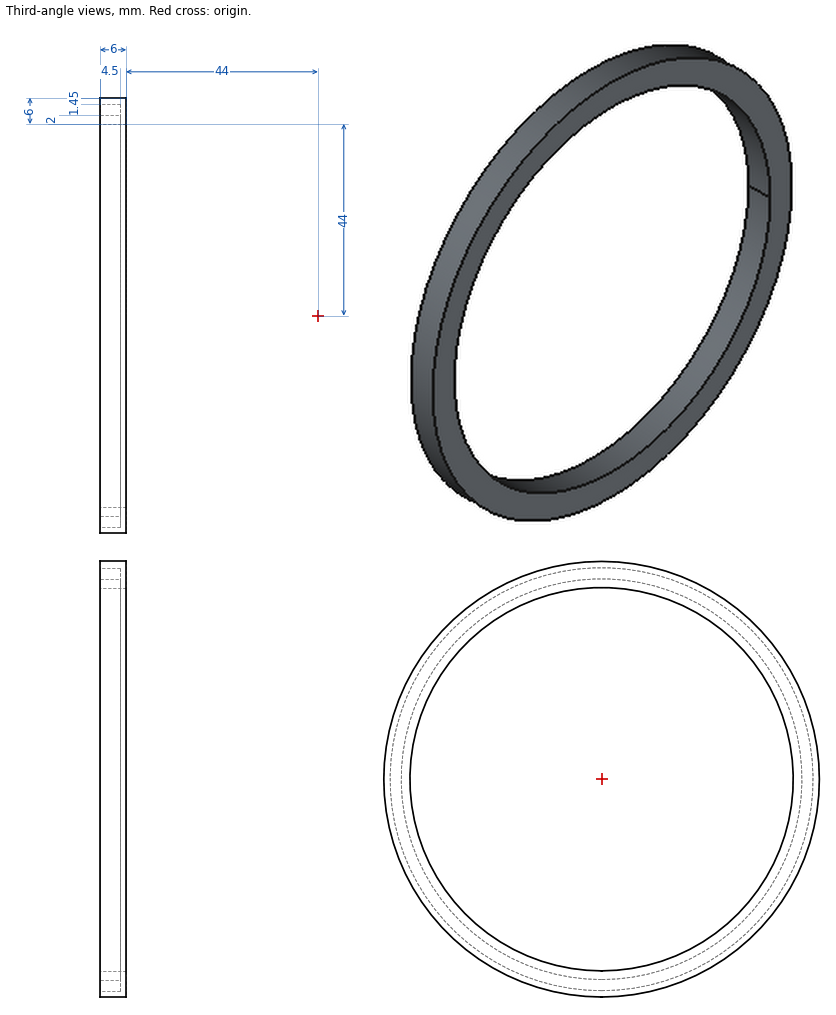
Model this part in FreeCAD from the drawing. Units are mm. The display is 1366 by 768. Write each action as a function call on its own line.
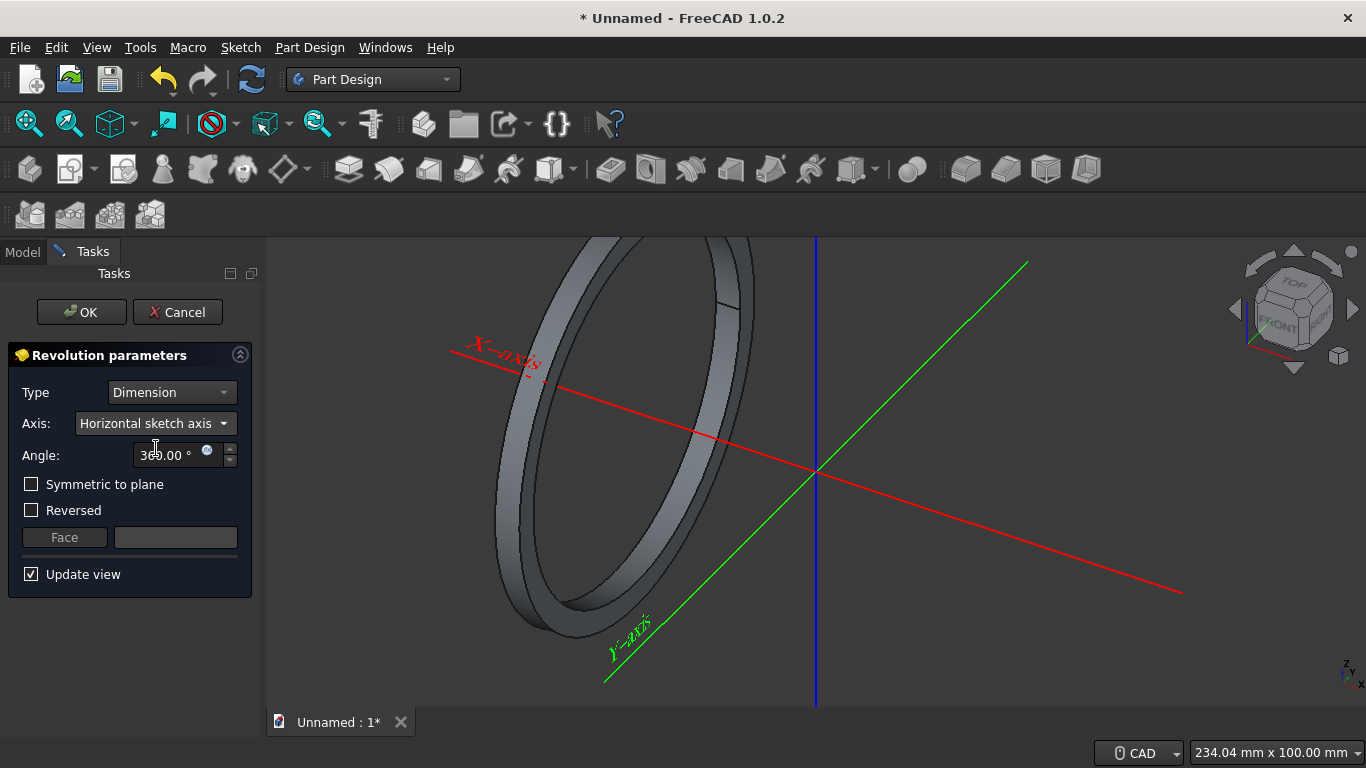
click(82, 312)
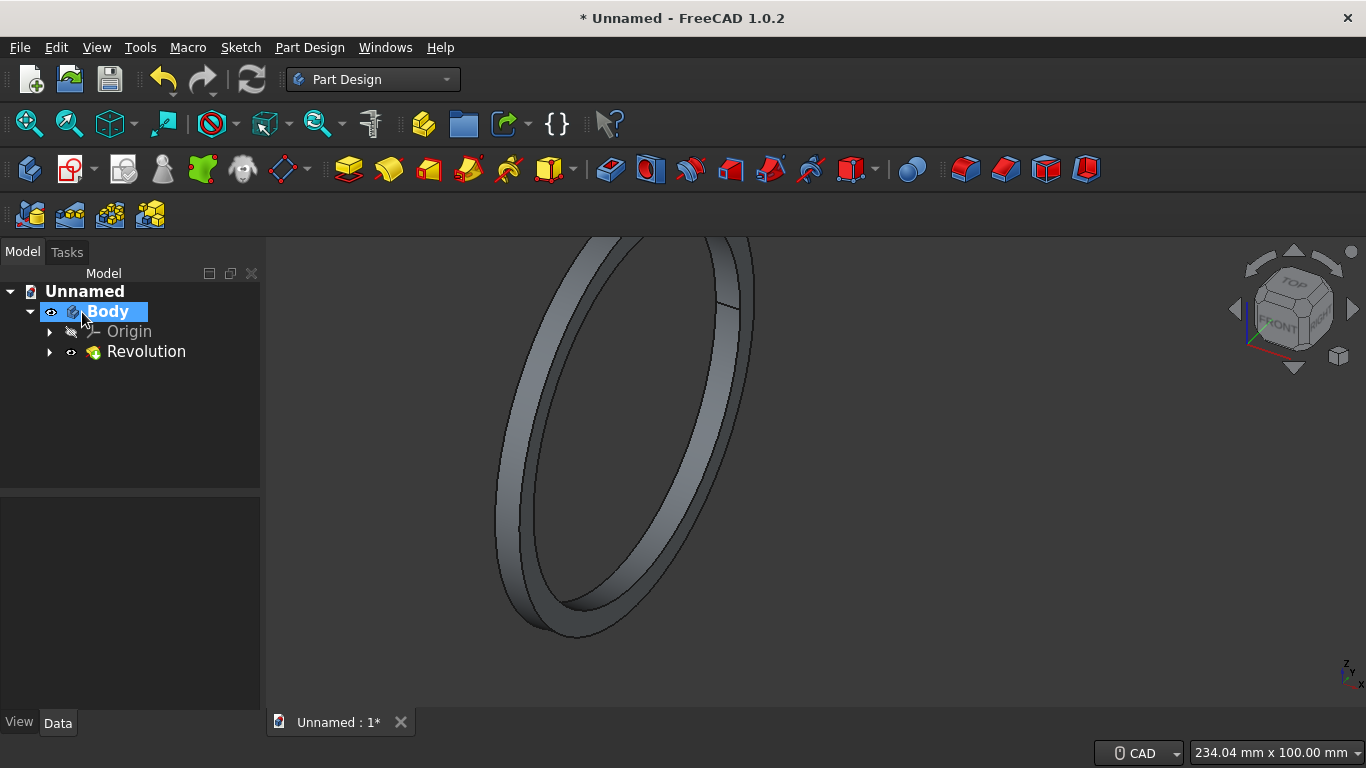
key(0)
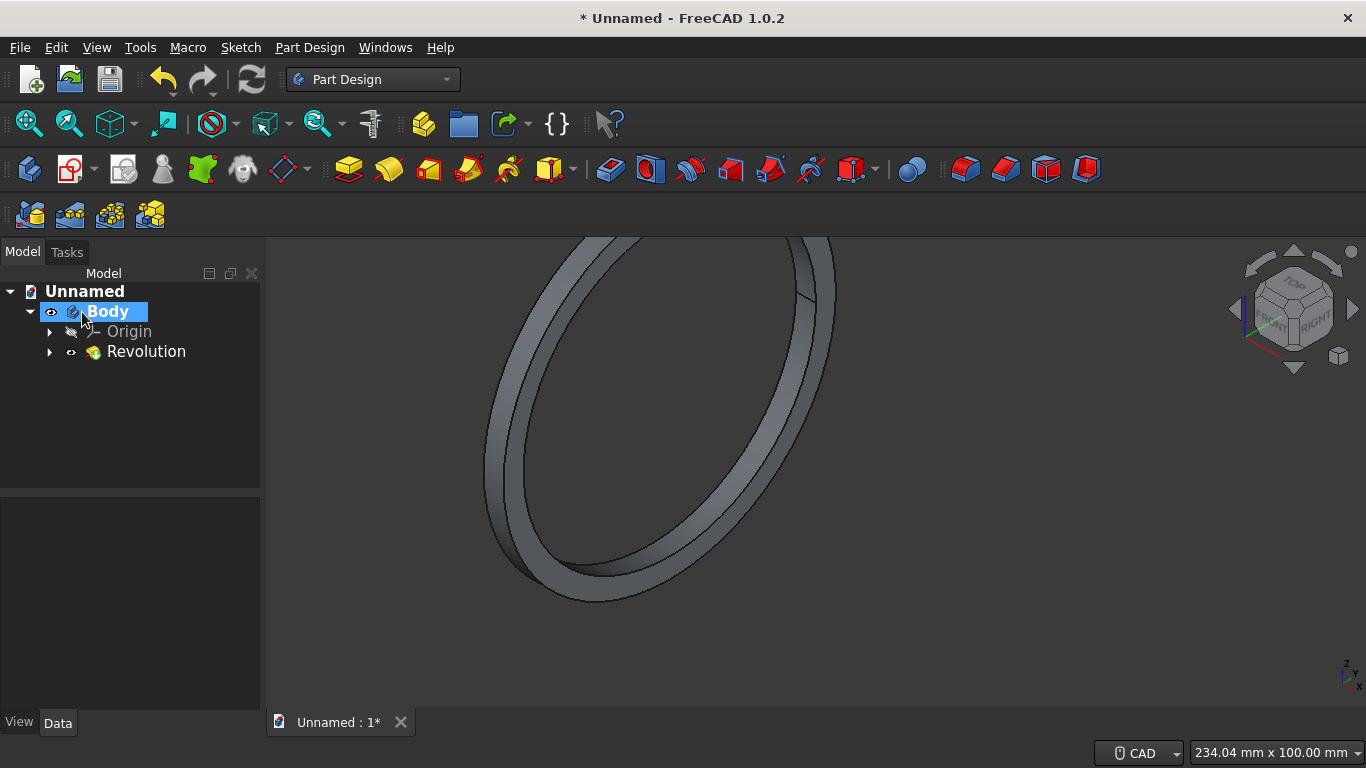
click(30, 124)